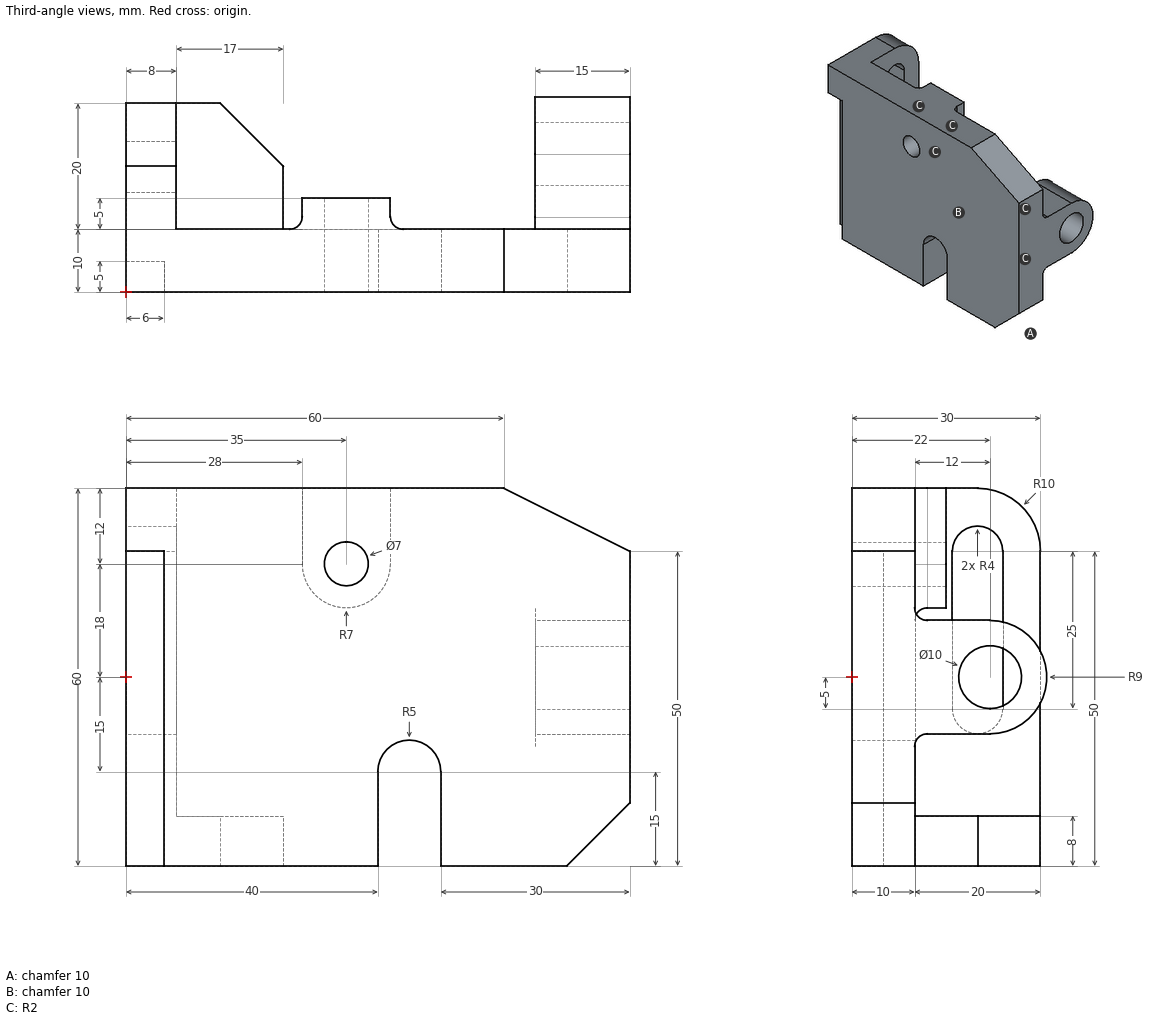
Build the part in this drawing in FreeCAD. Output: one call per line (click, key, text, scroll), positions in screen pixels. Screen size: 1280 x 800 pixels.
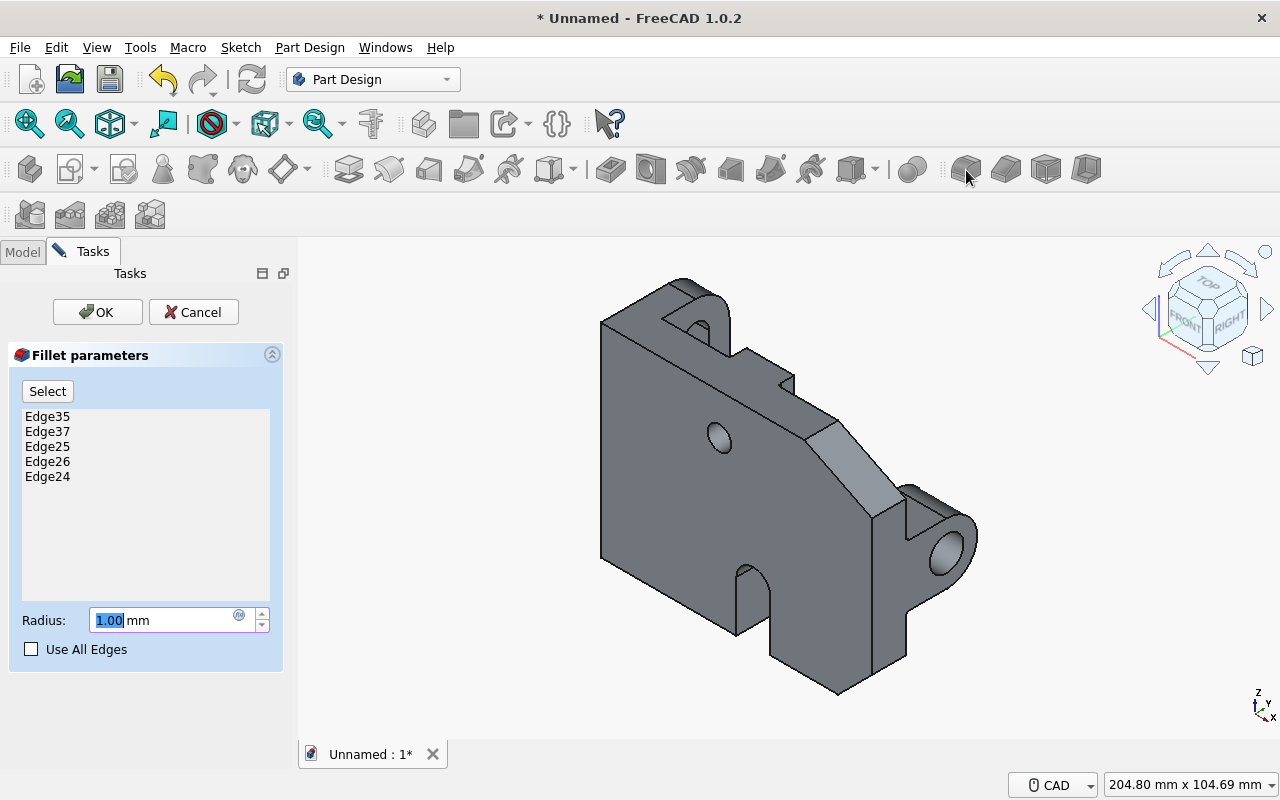
text(2)
key(Tab)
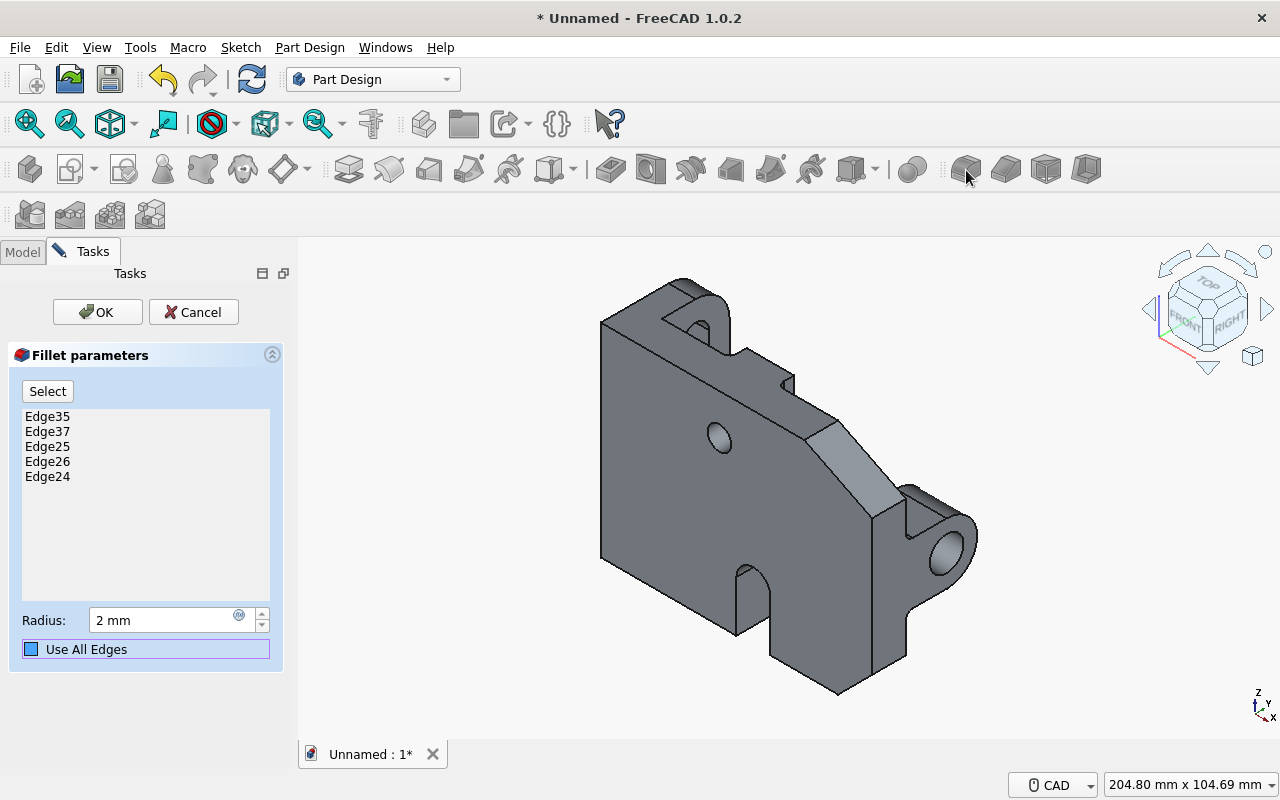
click(98, 312)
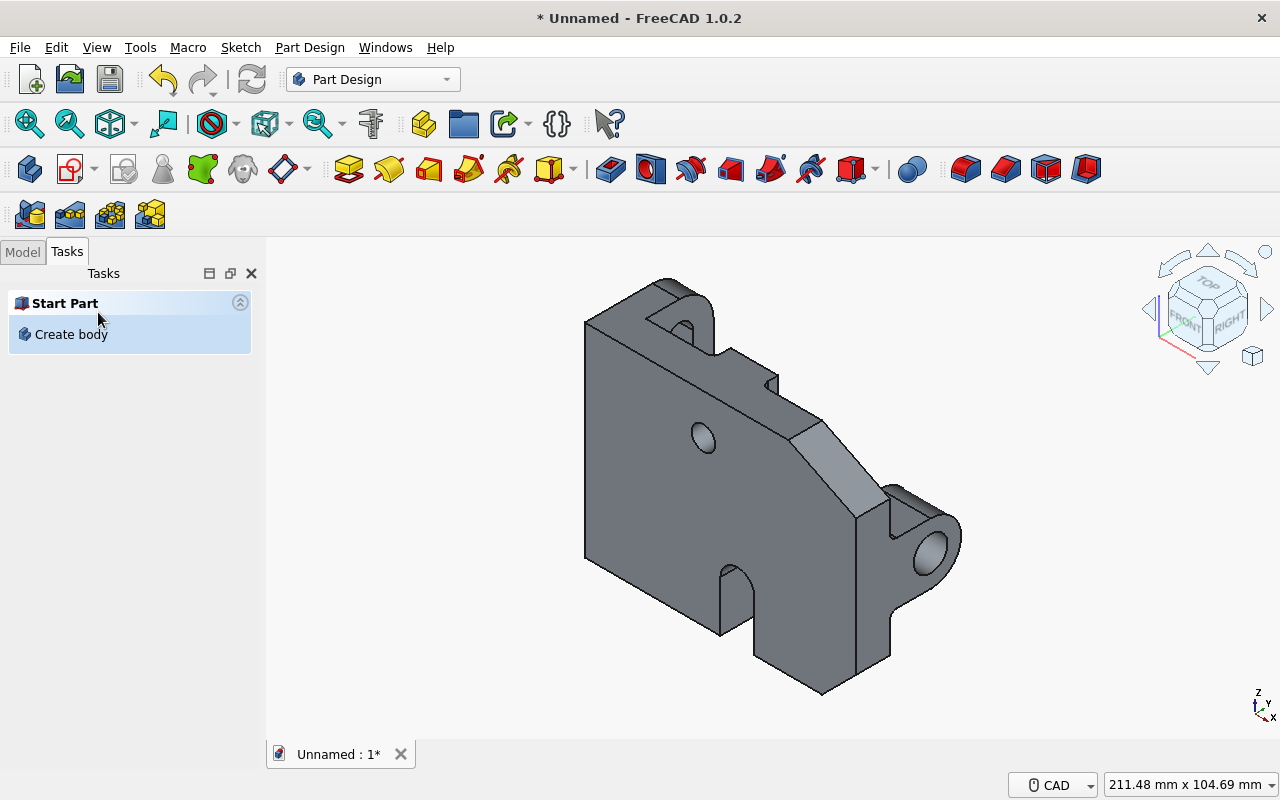
key(5)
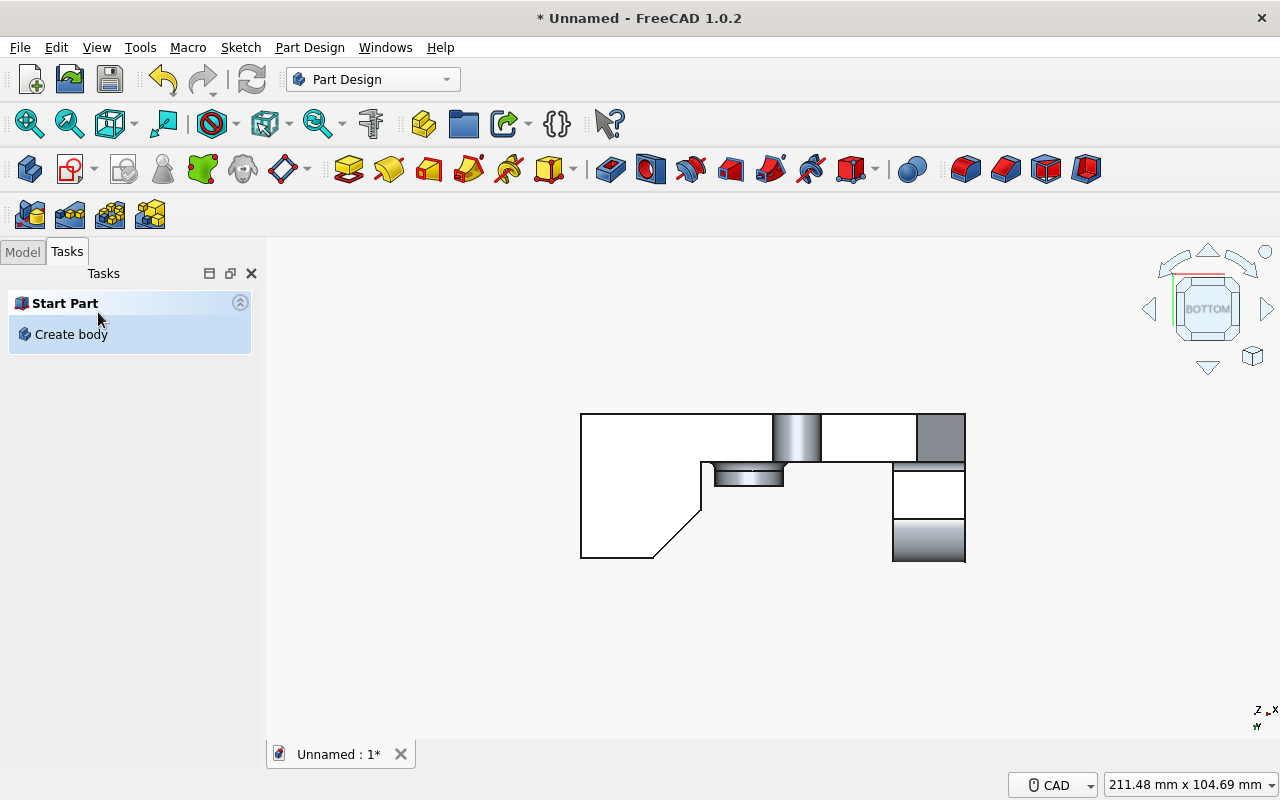
click(30, 124)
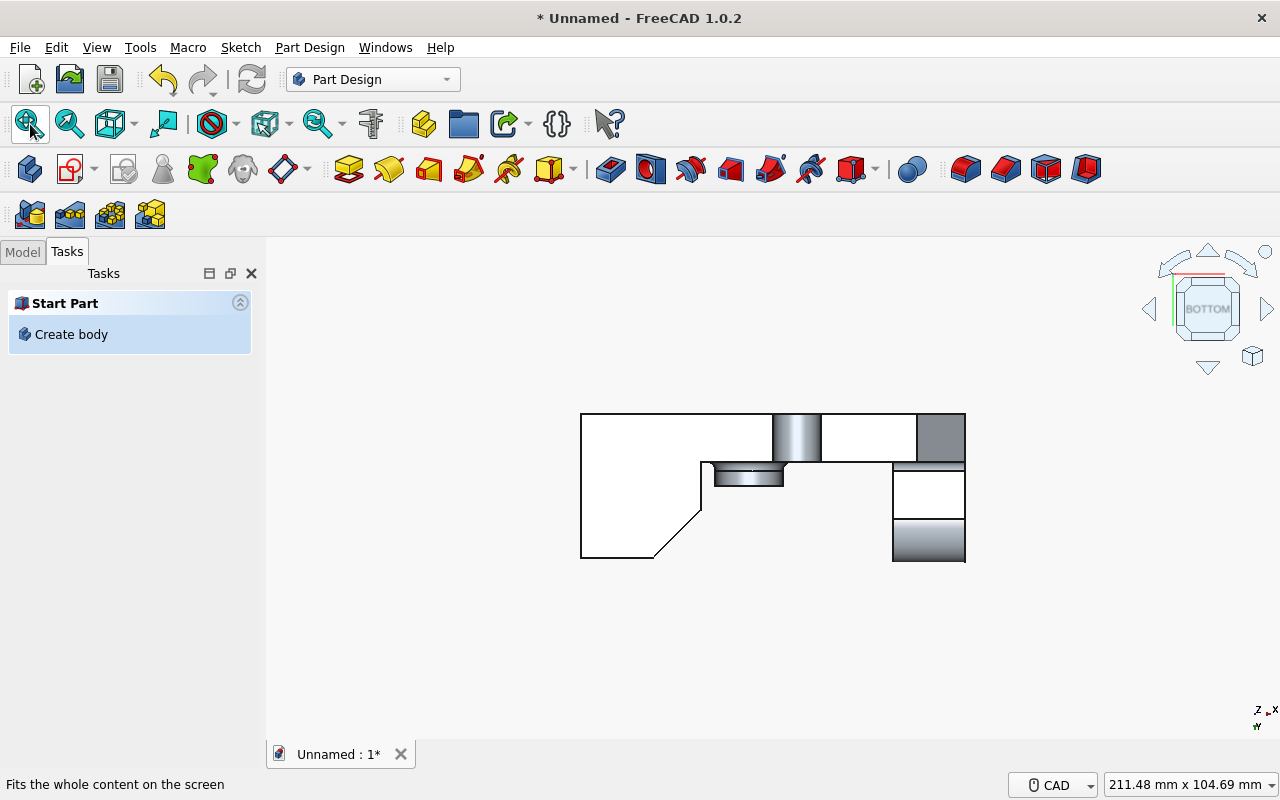
click(650, 485)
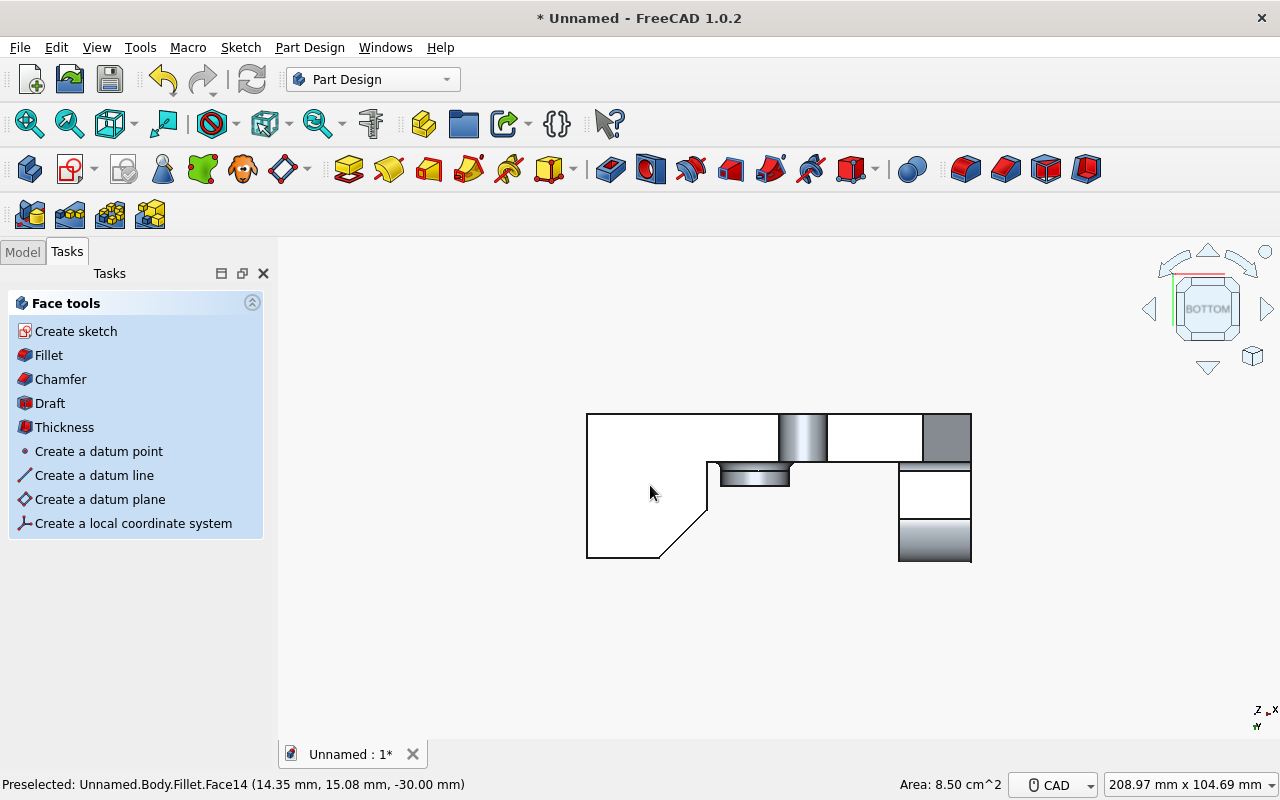
click(70, 170)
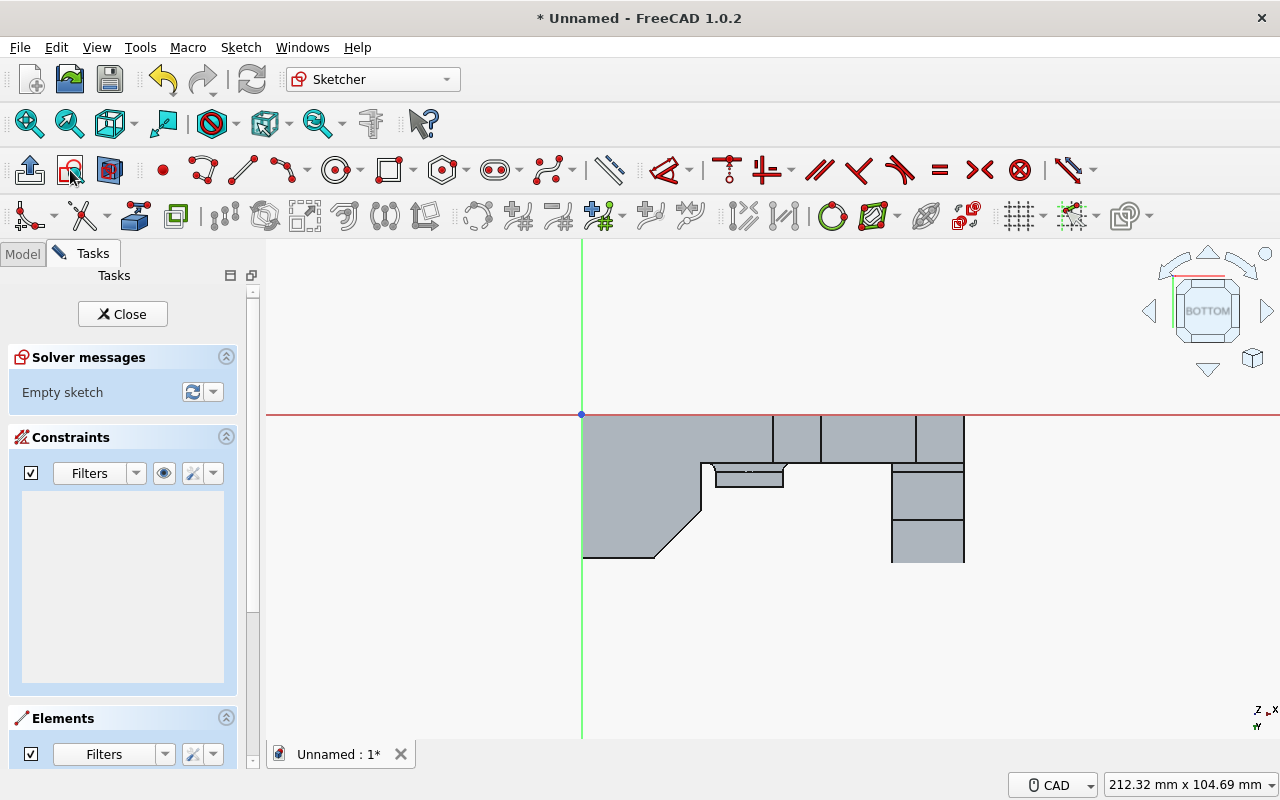
scroll(588, 422, up, 13)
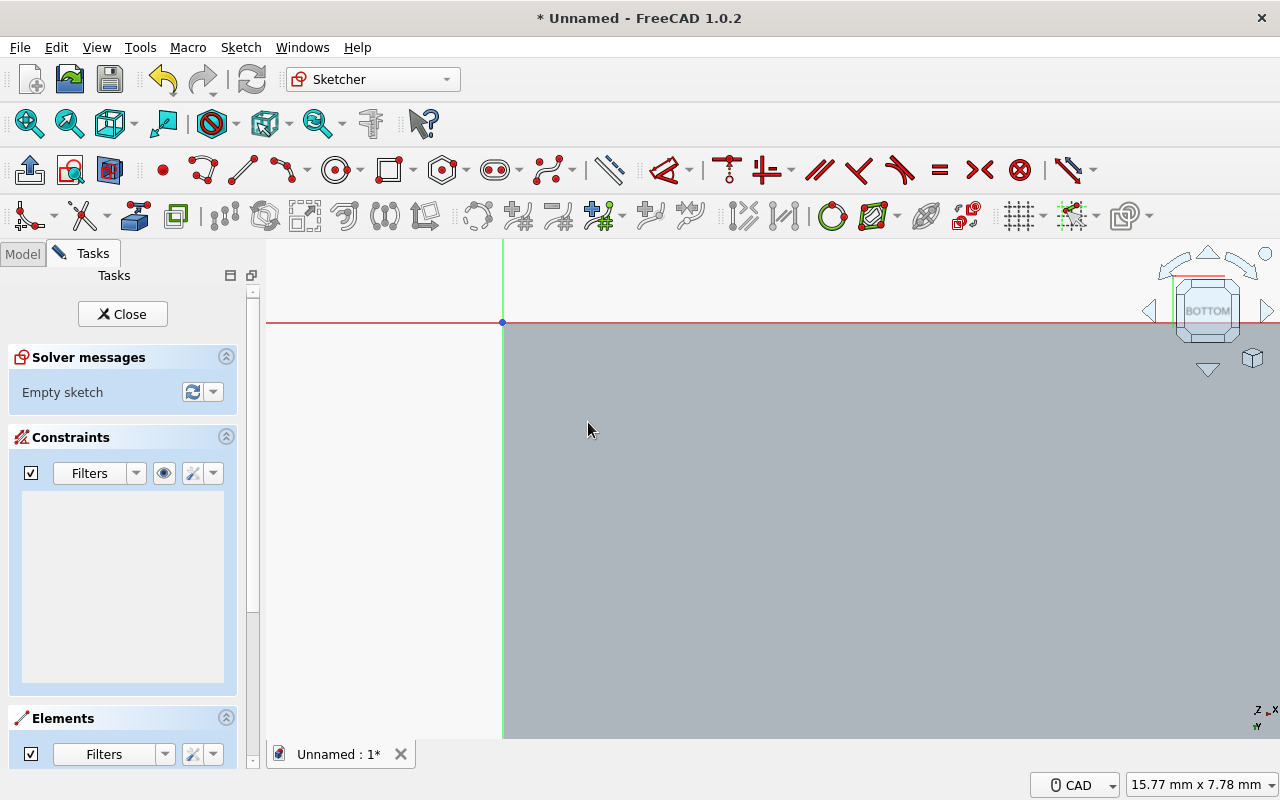
click(390, 170)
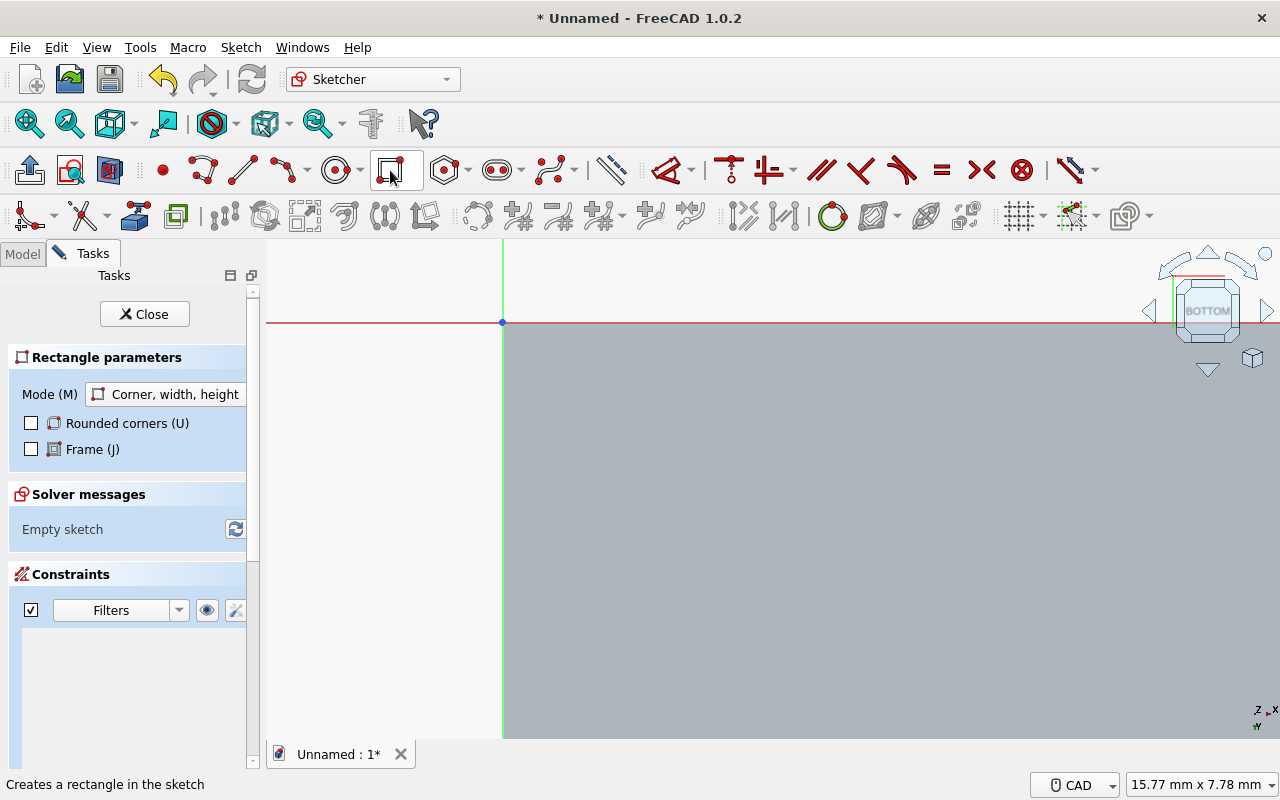
click(503, 323)
click(889, 644)
key(Escape)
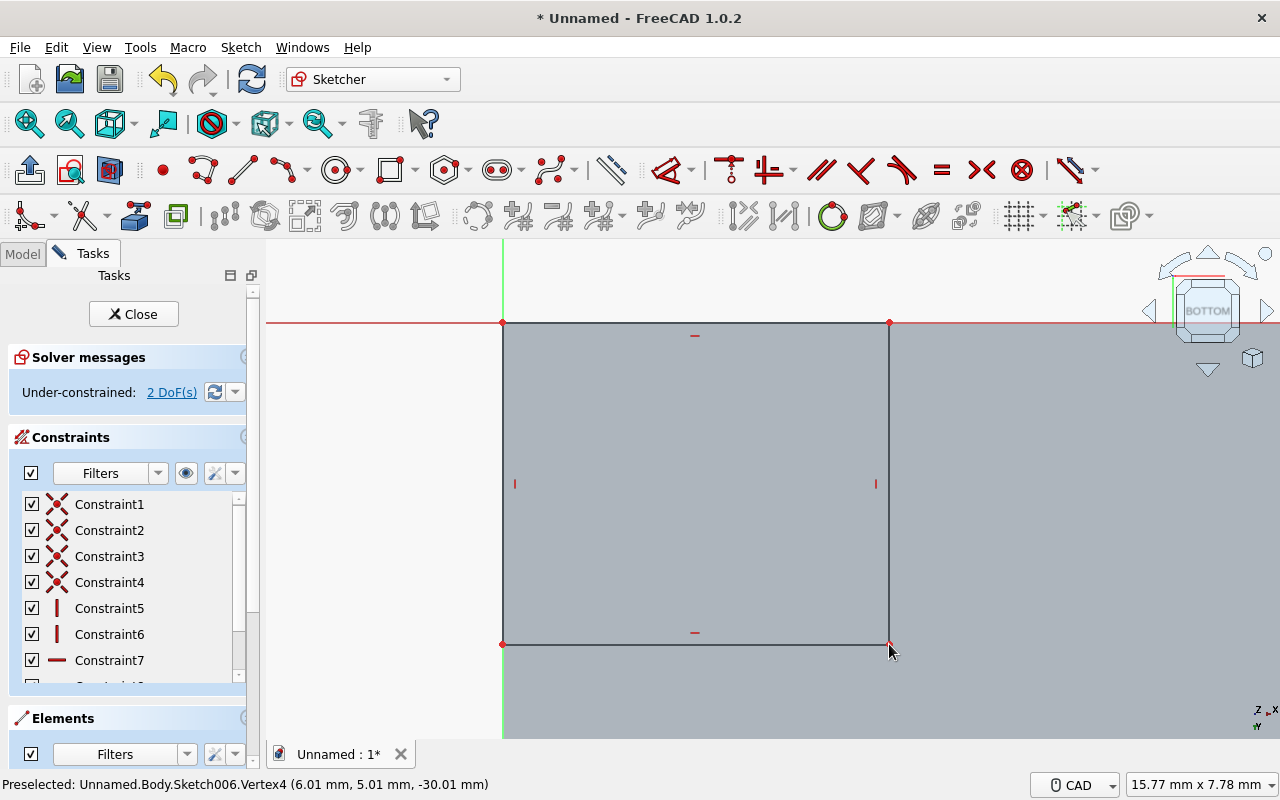
click(666, 170)